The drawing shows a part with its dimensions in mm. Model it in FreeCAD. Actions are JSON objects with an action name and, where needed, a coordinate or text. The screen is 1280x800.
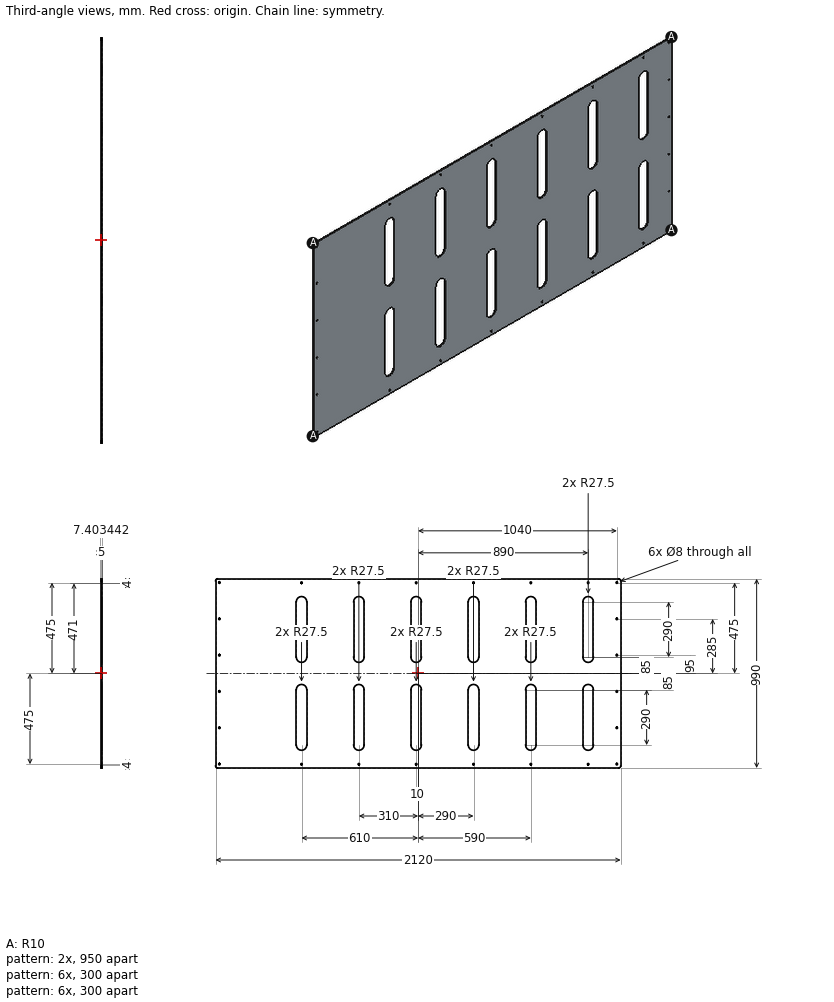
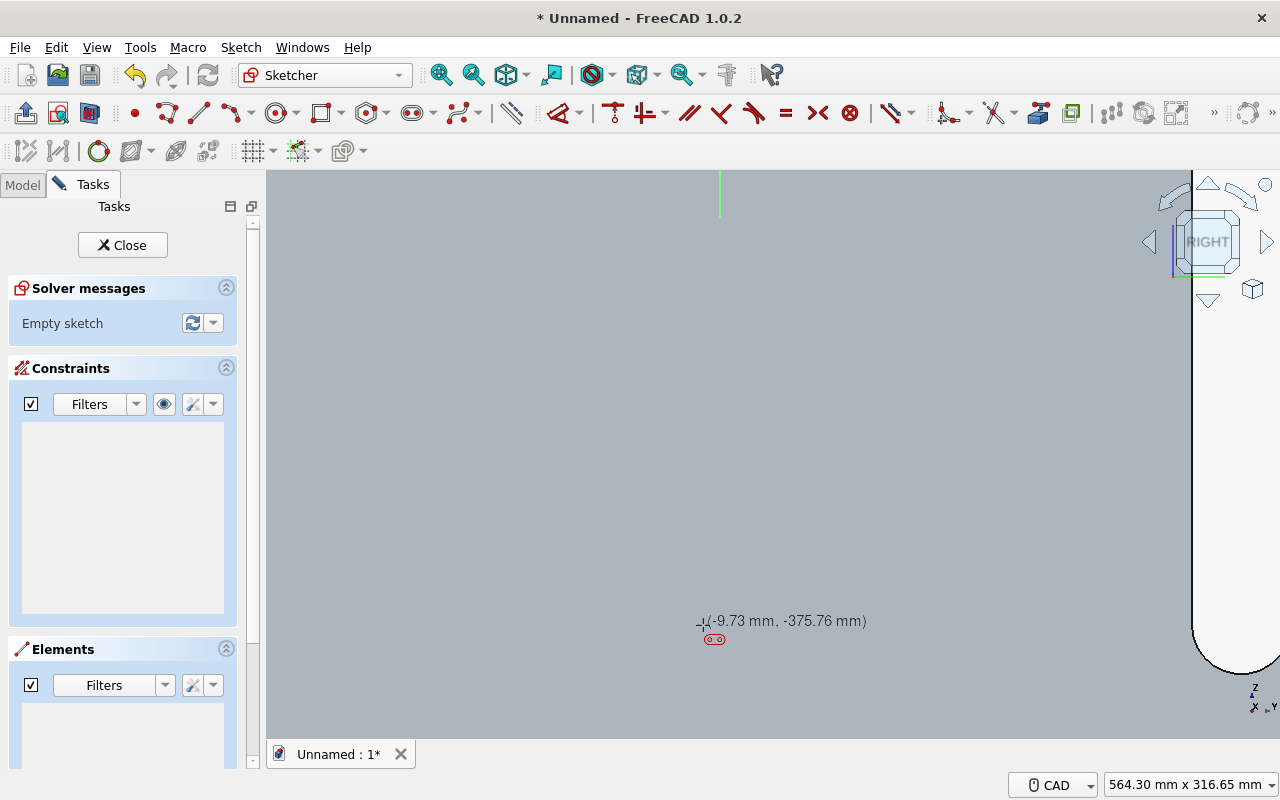
{"action": "left_click", "coordinate": [702, 625]}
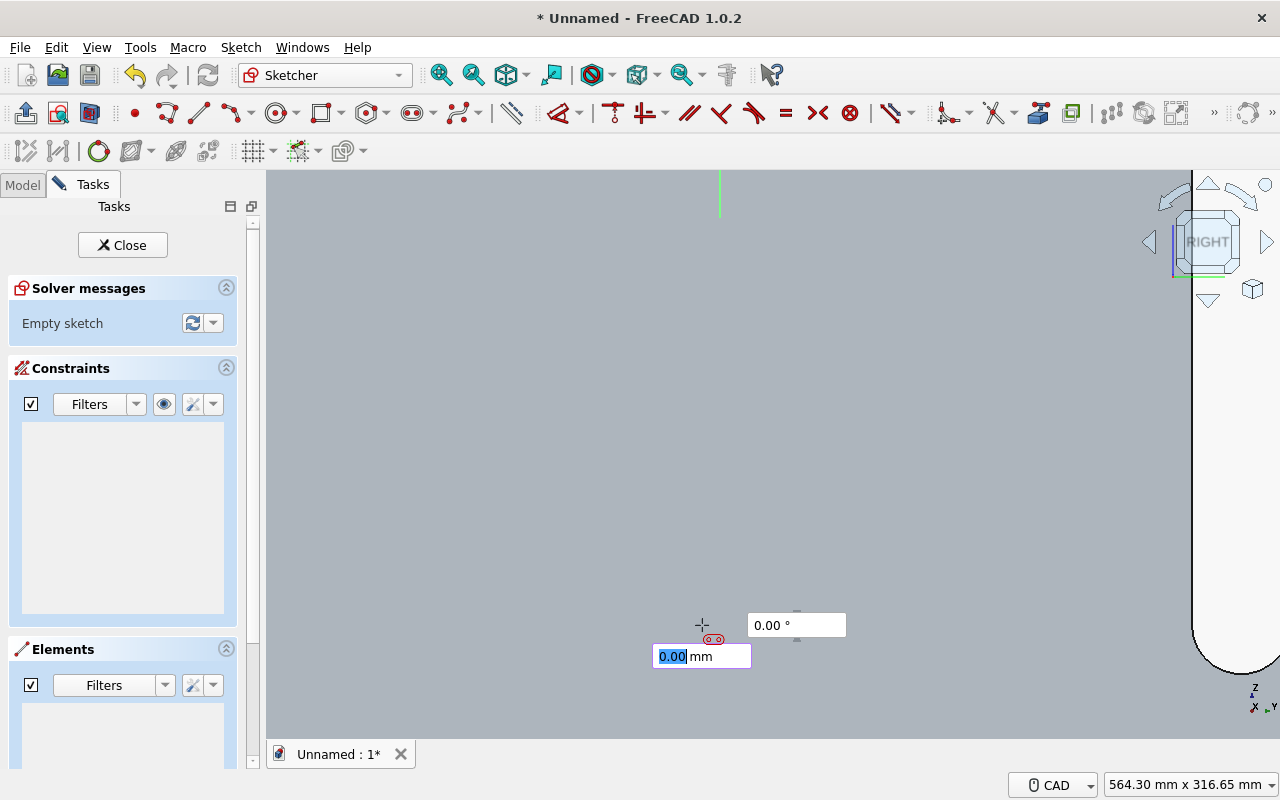
{"action": "scroll", "coordinate": [707, 627], "scroll_direction": "down", "scroll_amount": 3}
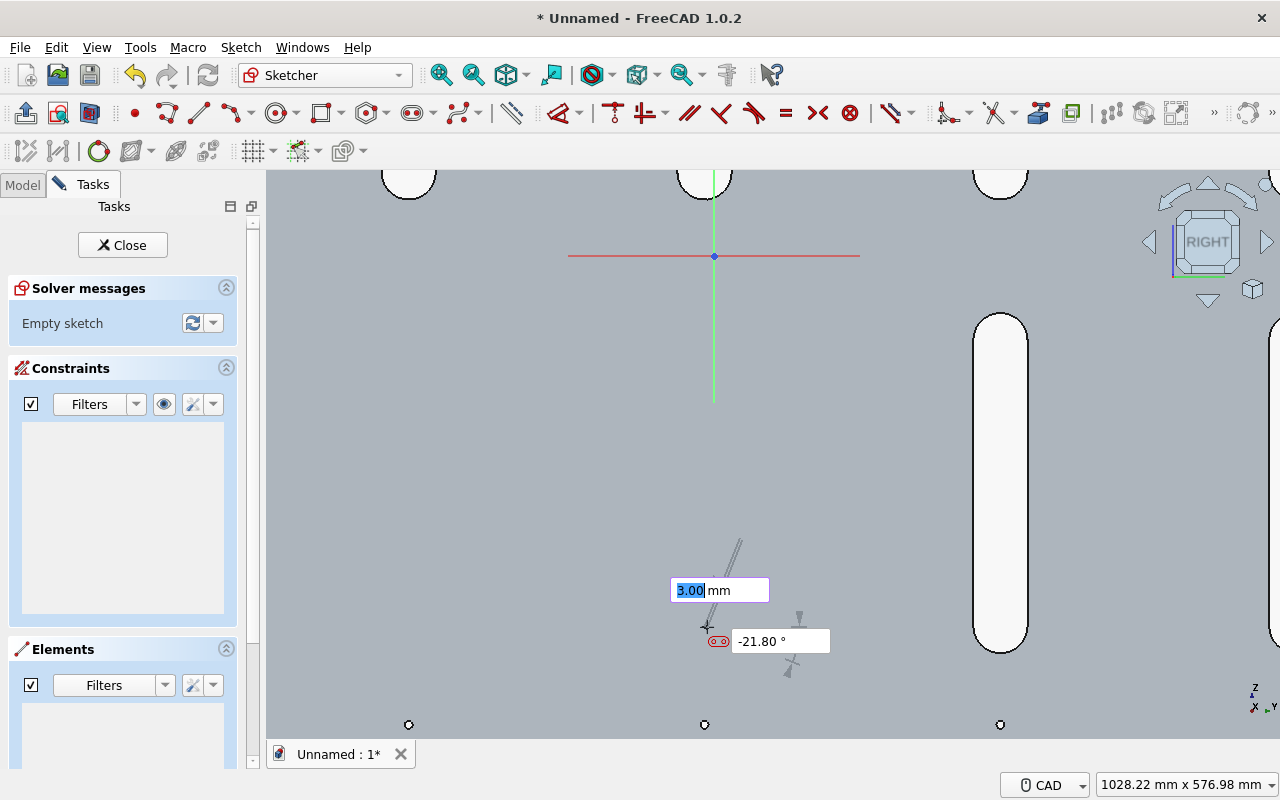
{"action": "scroll", "coordinate": [705, 340], "scroll_direction": "up", "scroll_amount": 3}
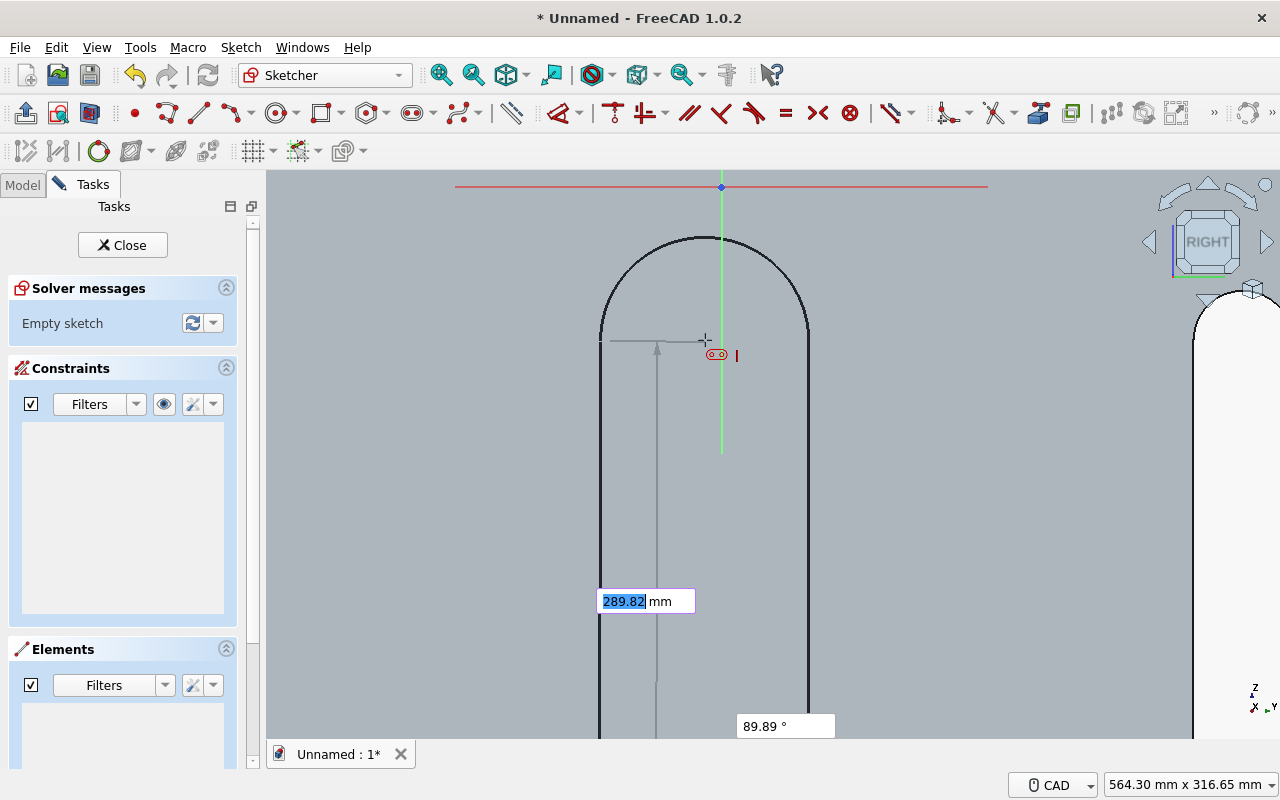
{"action": "left_click", "coordinate": [704, 340]}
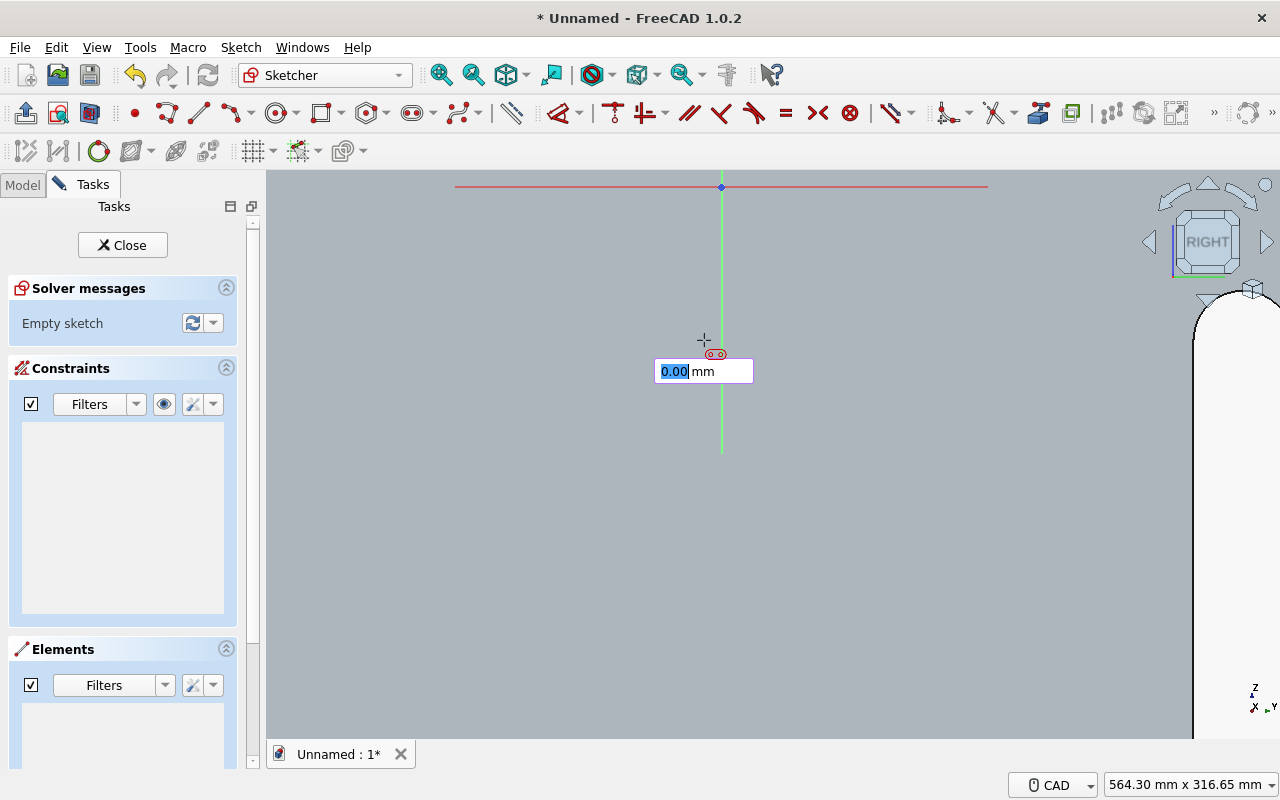
{"action": "left_click", "coordinate": [753, 601]}
{"action": "key", "text": "Escape"}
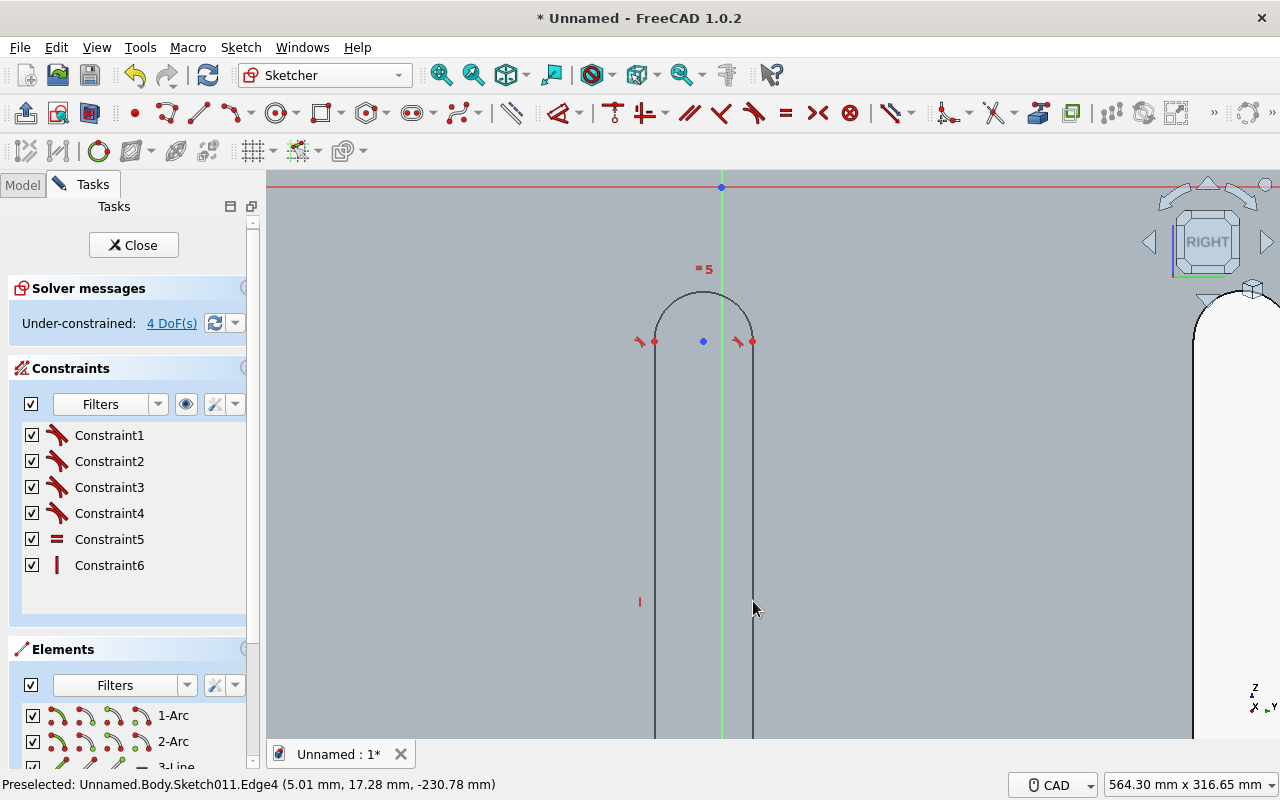
{"action": "left_click", "coordinate": [558, 114]}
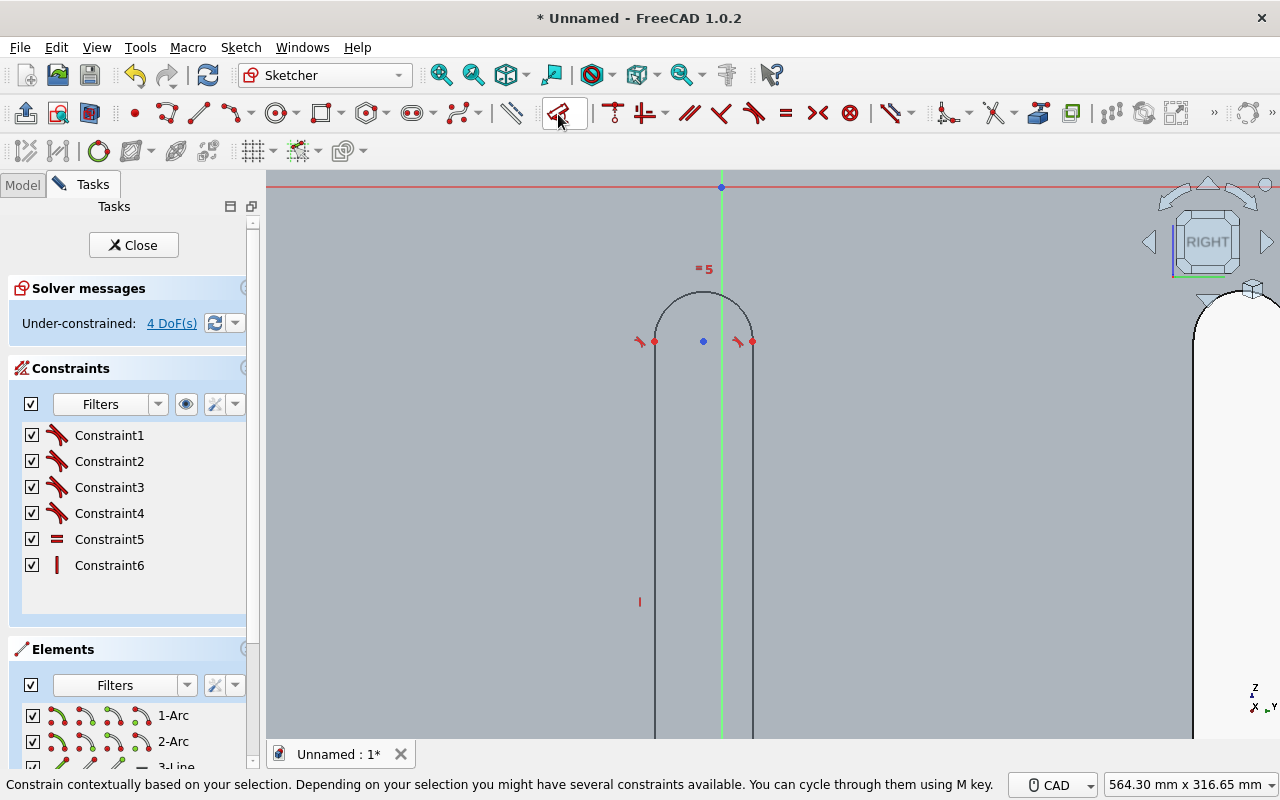
{"action": "scroll", "coordinate": [705, 340], "scroll_direction": "down", "scroll_amount": 3}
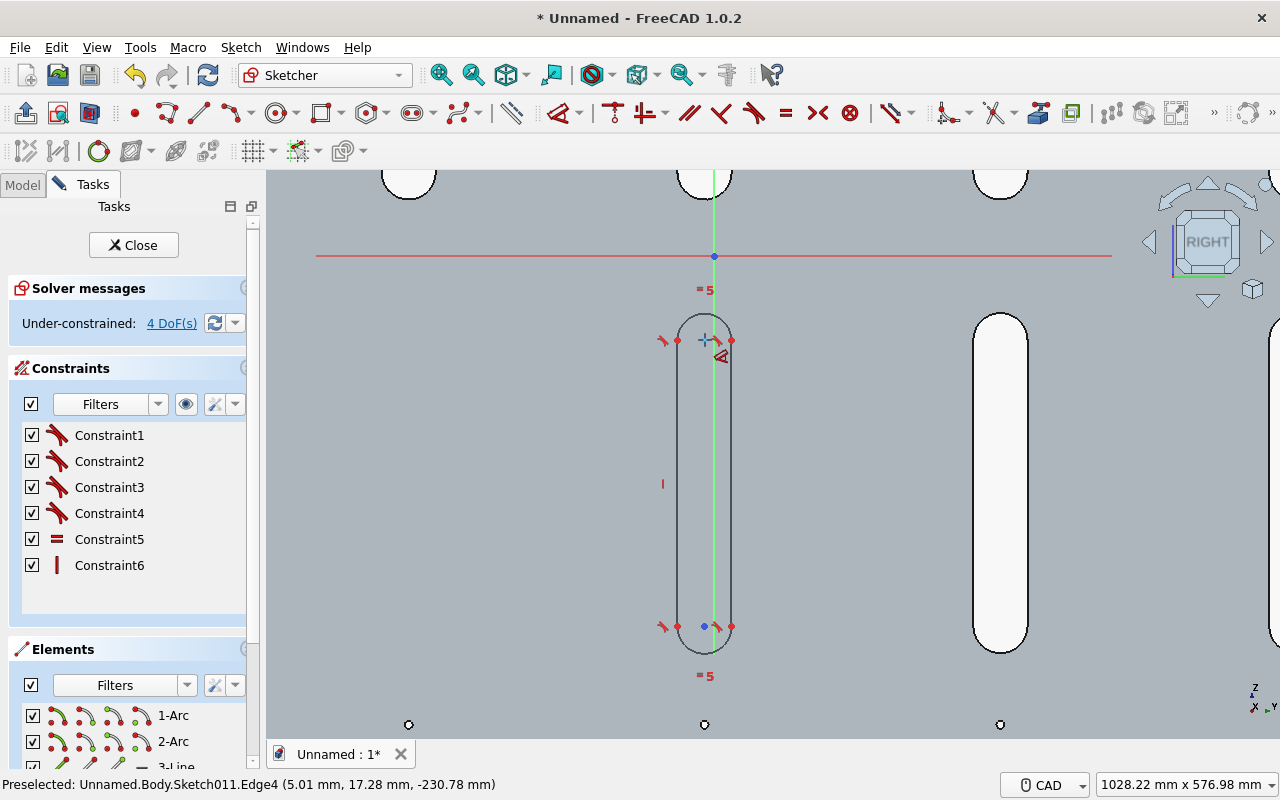
{"action": "scroll", "coordinate": [689, 649], "scroll_direction": "up", "scroll_amount": 2}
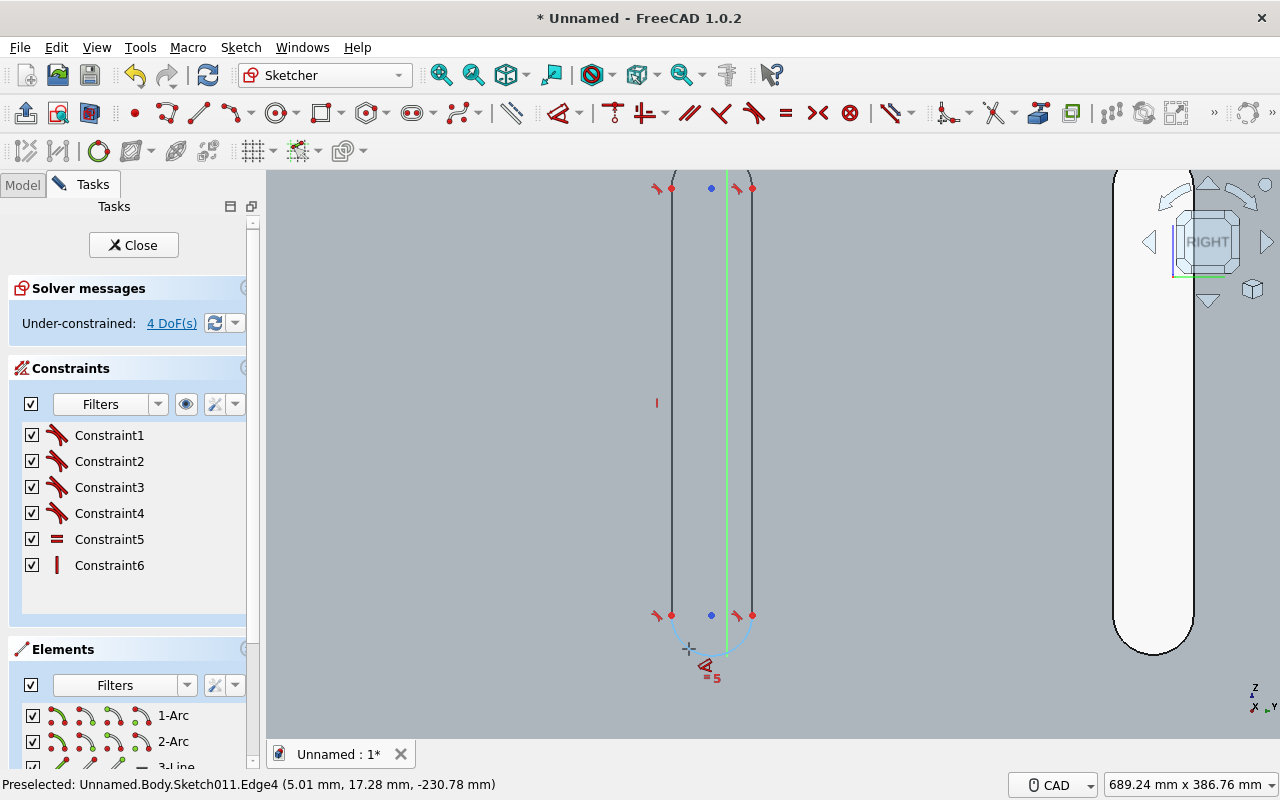
{"action": "left_click", "coordinate": [688, 648]}
{"action": "left_click", "coordinate": [669, 674]}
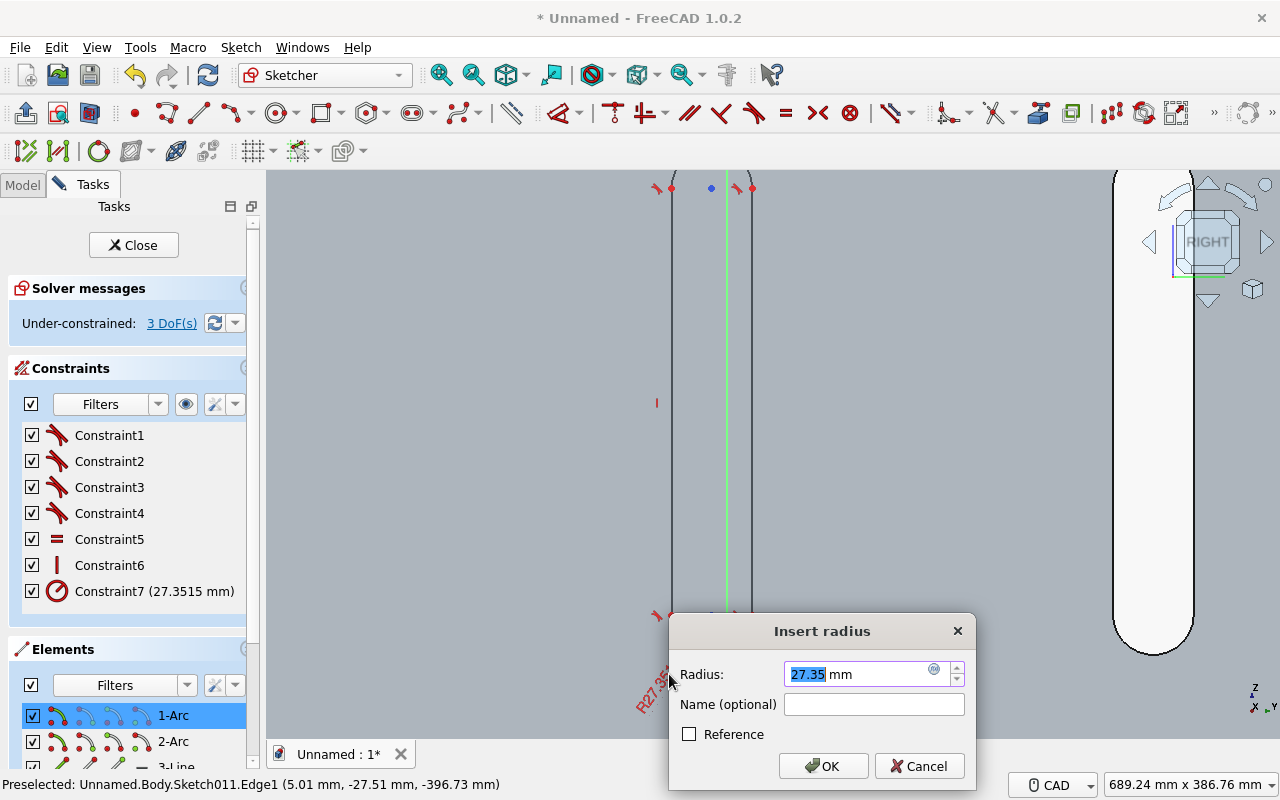
{"action": "type", "text": "27.5"}
{"action": "key", "text": "Return"}